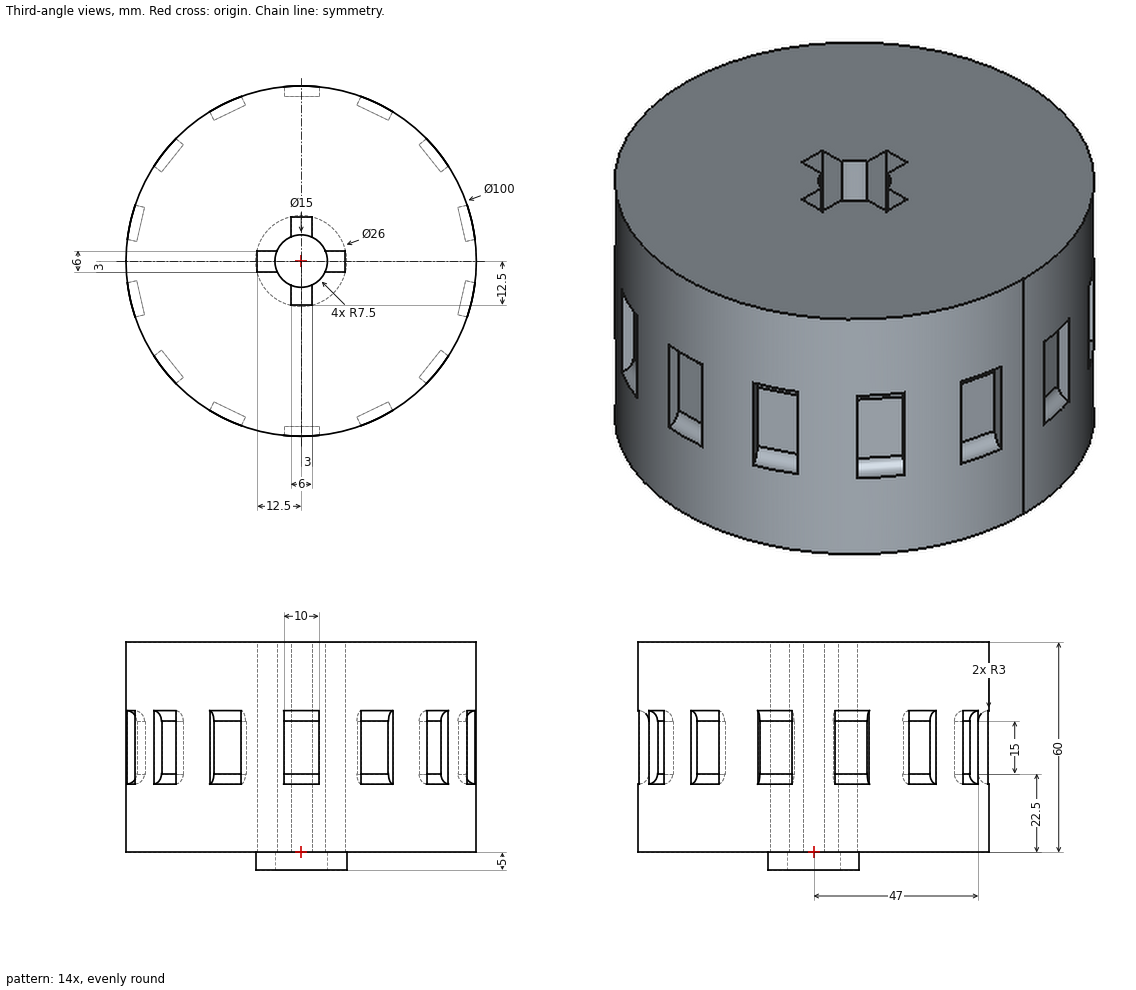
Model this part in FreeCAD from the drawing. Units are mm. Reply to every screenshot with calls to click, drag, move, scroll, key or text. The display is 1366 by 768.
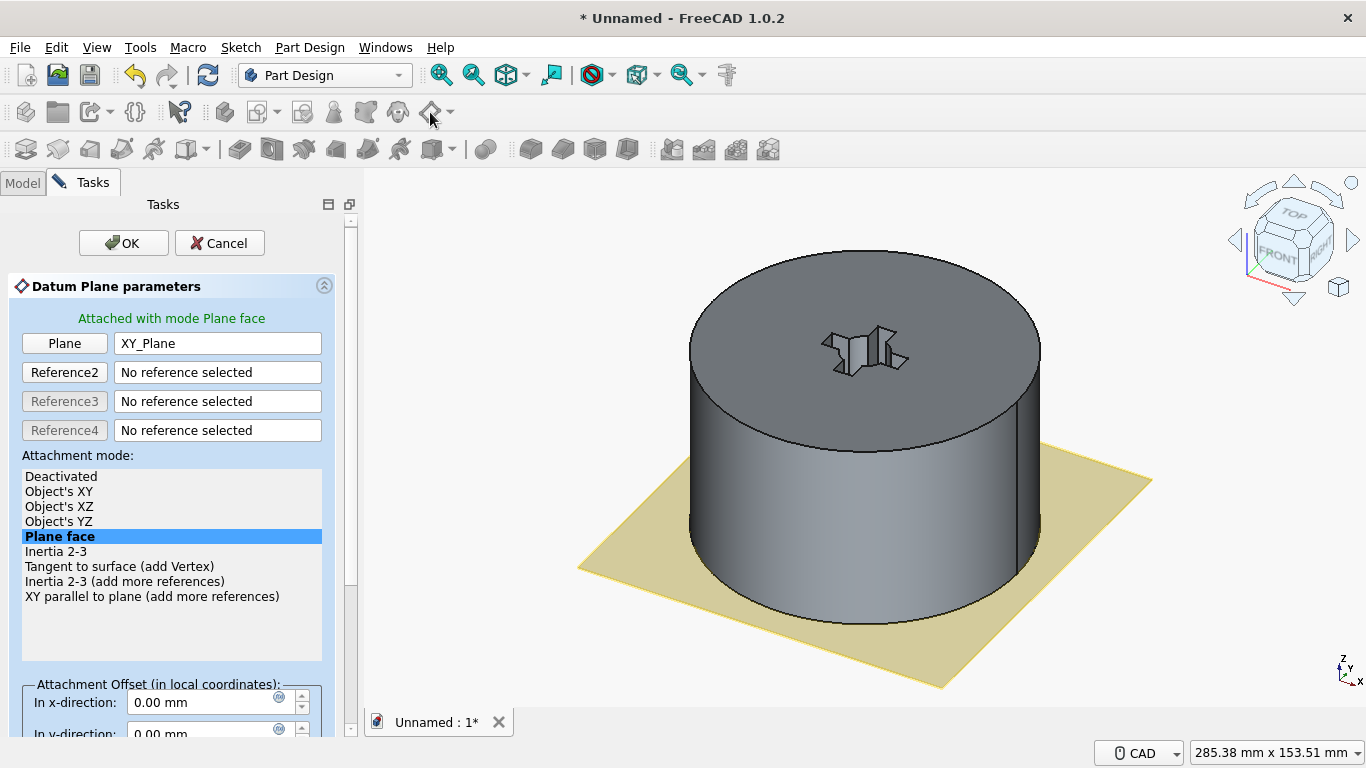
scroll(351, 475, down, 2)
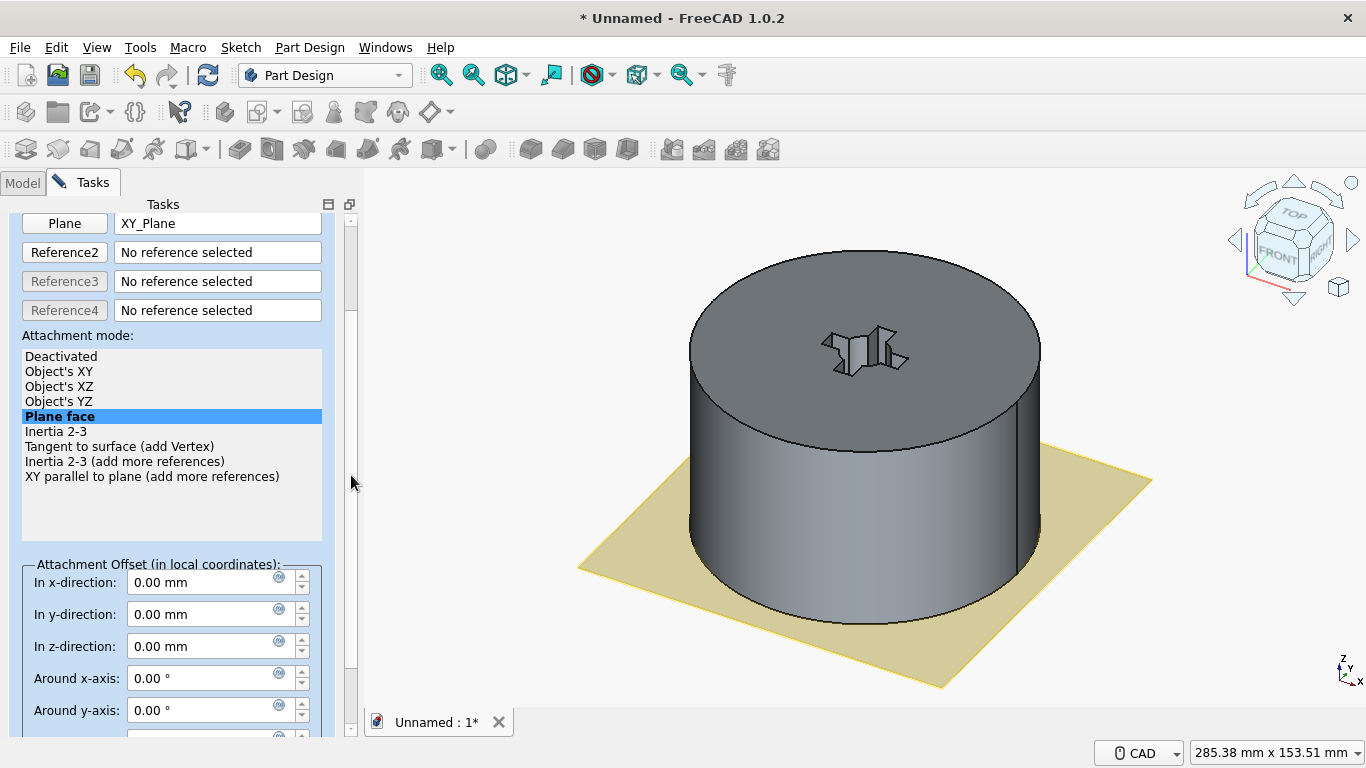
triple_click(210, 646)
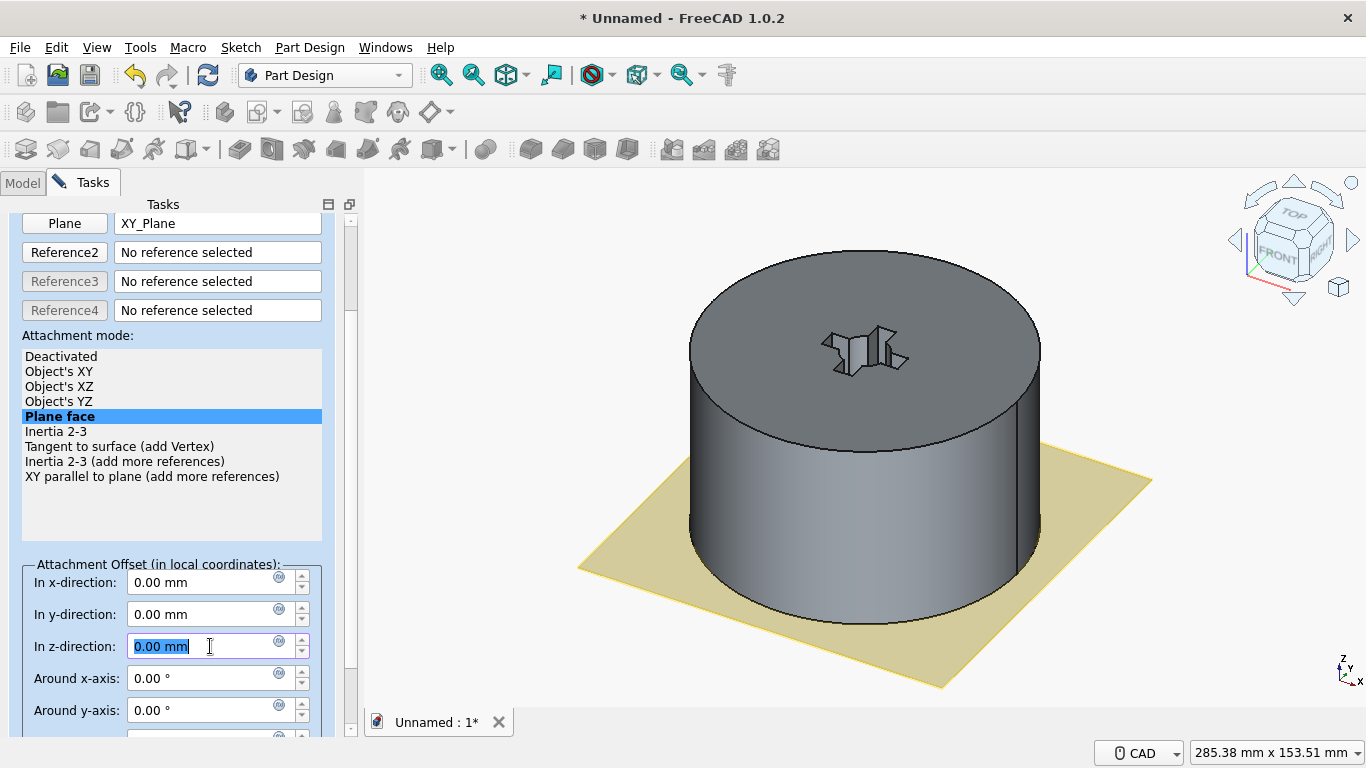
text(-5)
key(Tab)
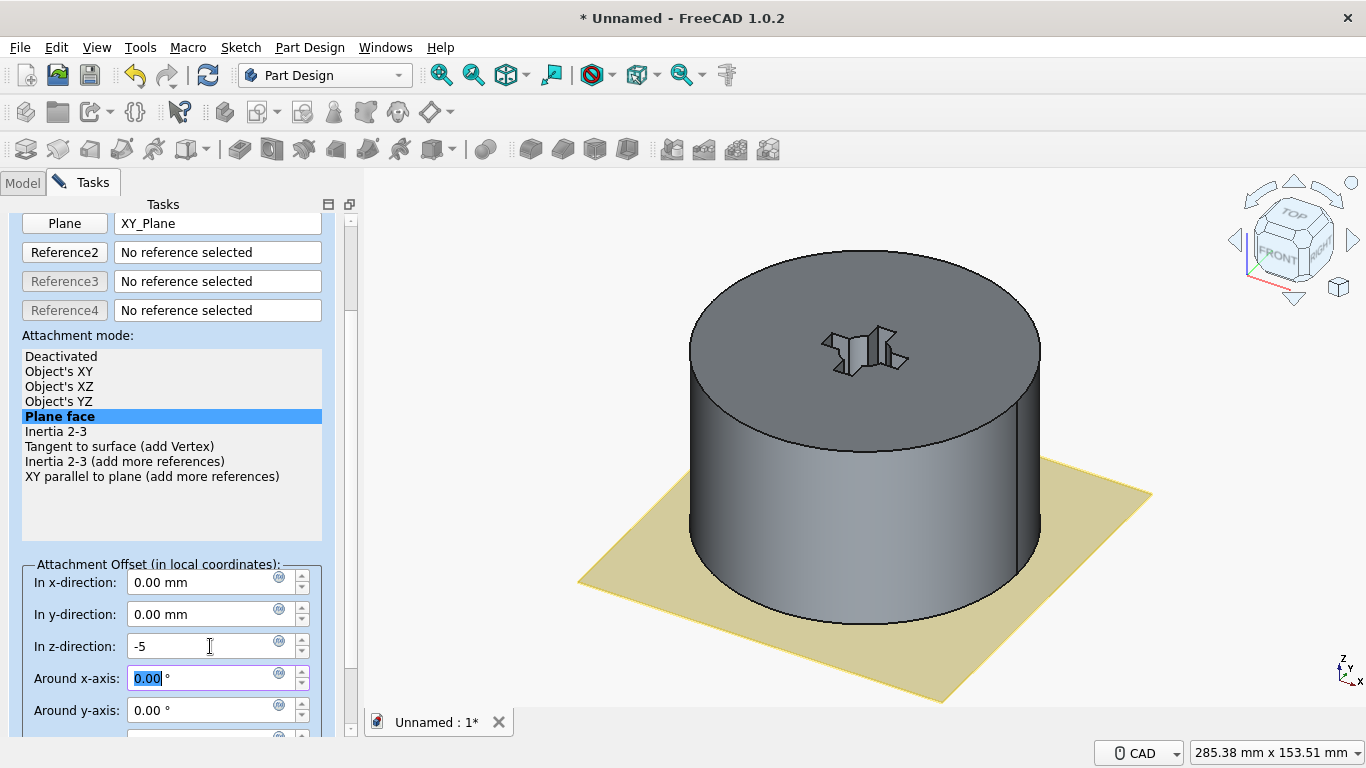
scroll(351, 475, up, 3)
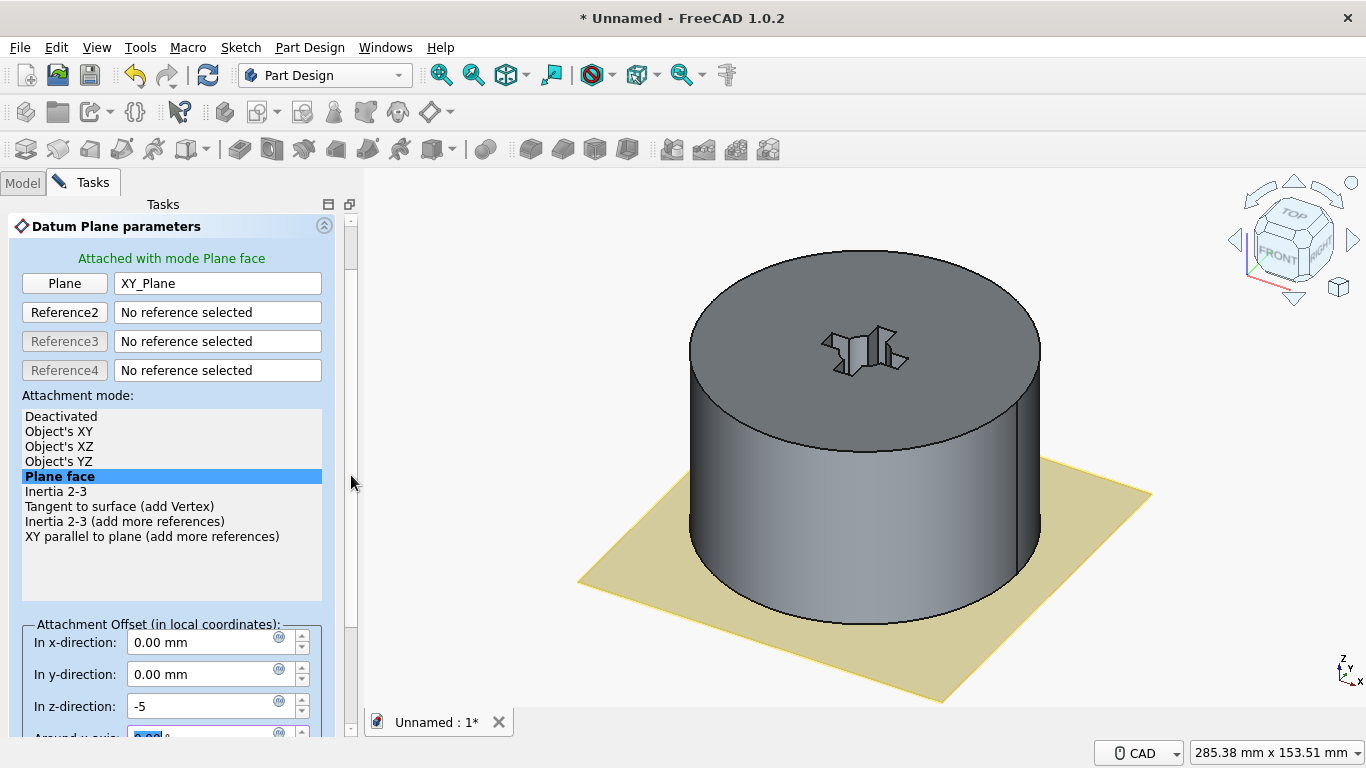
click(124, 243)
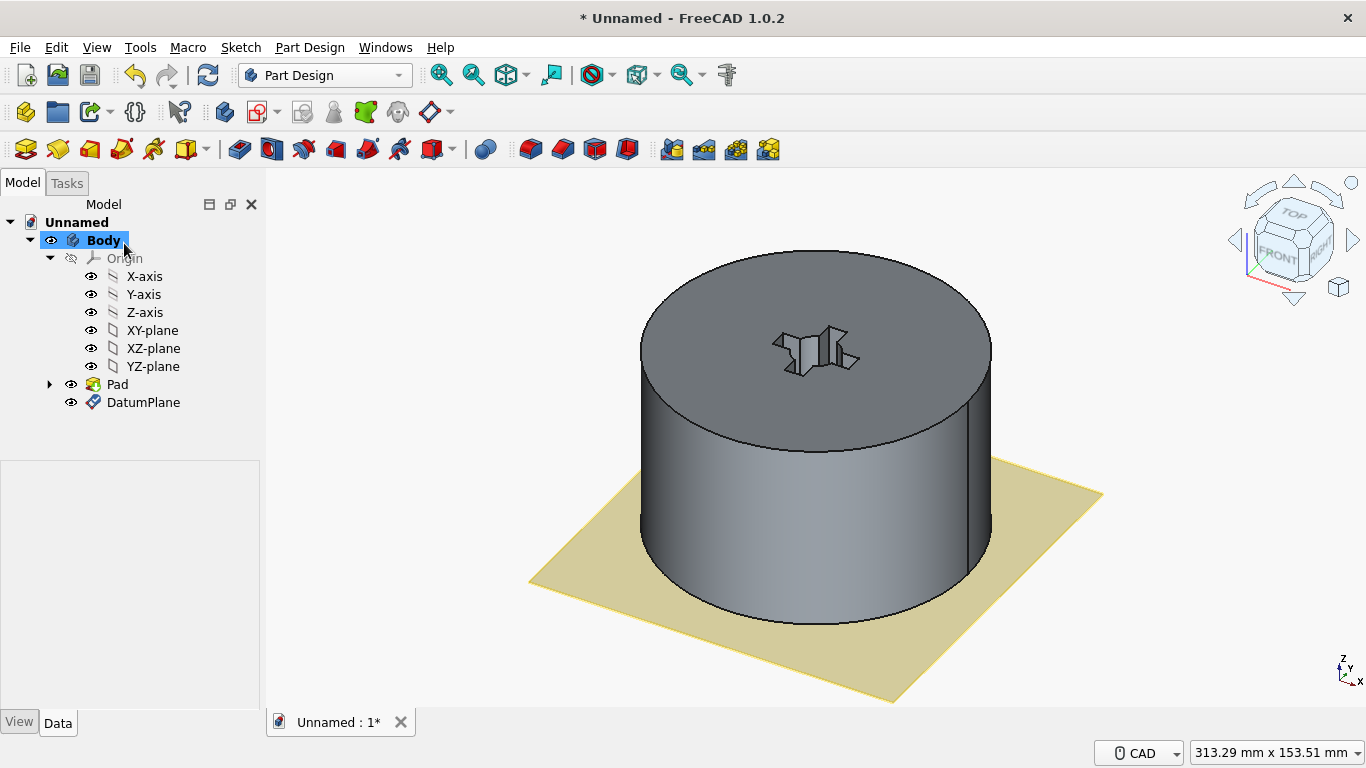
click(116, 402)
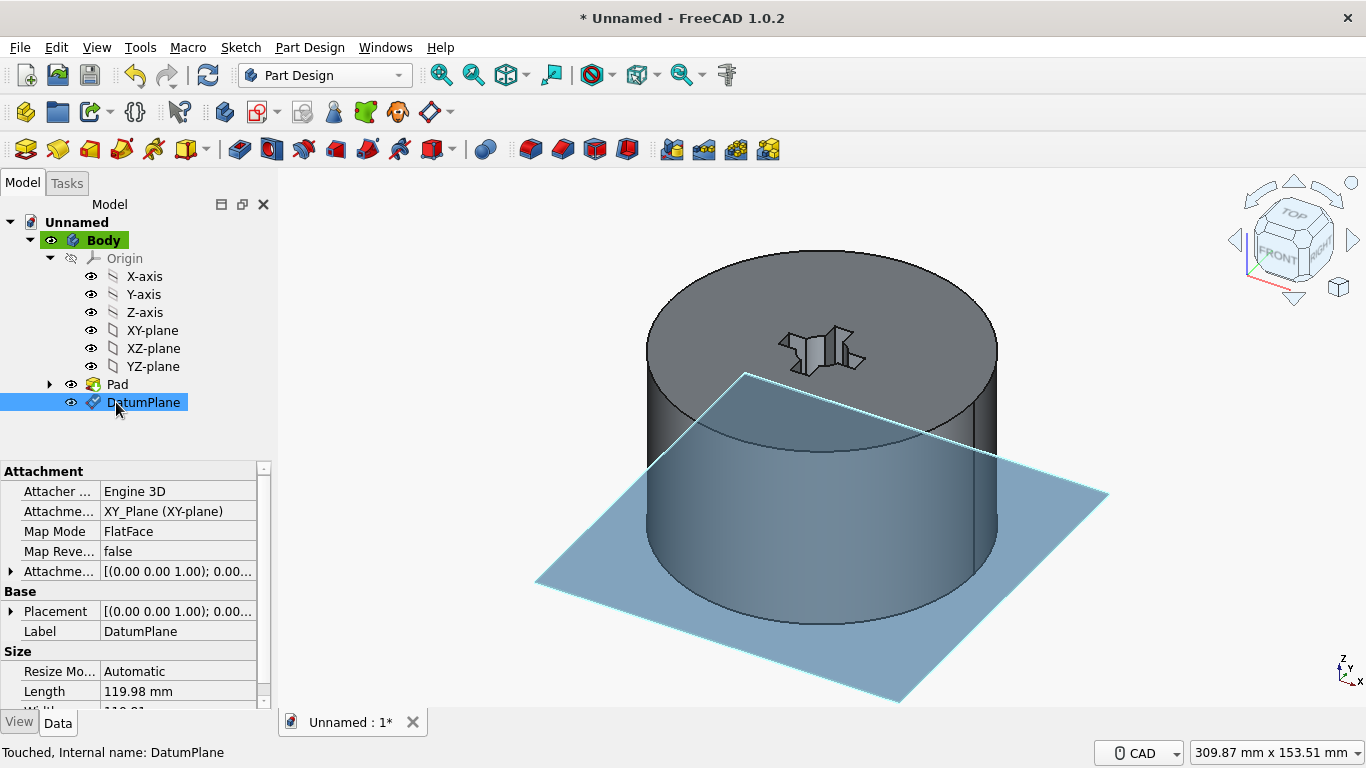
click(258, 112)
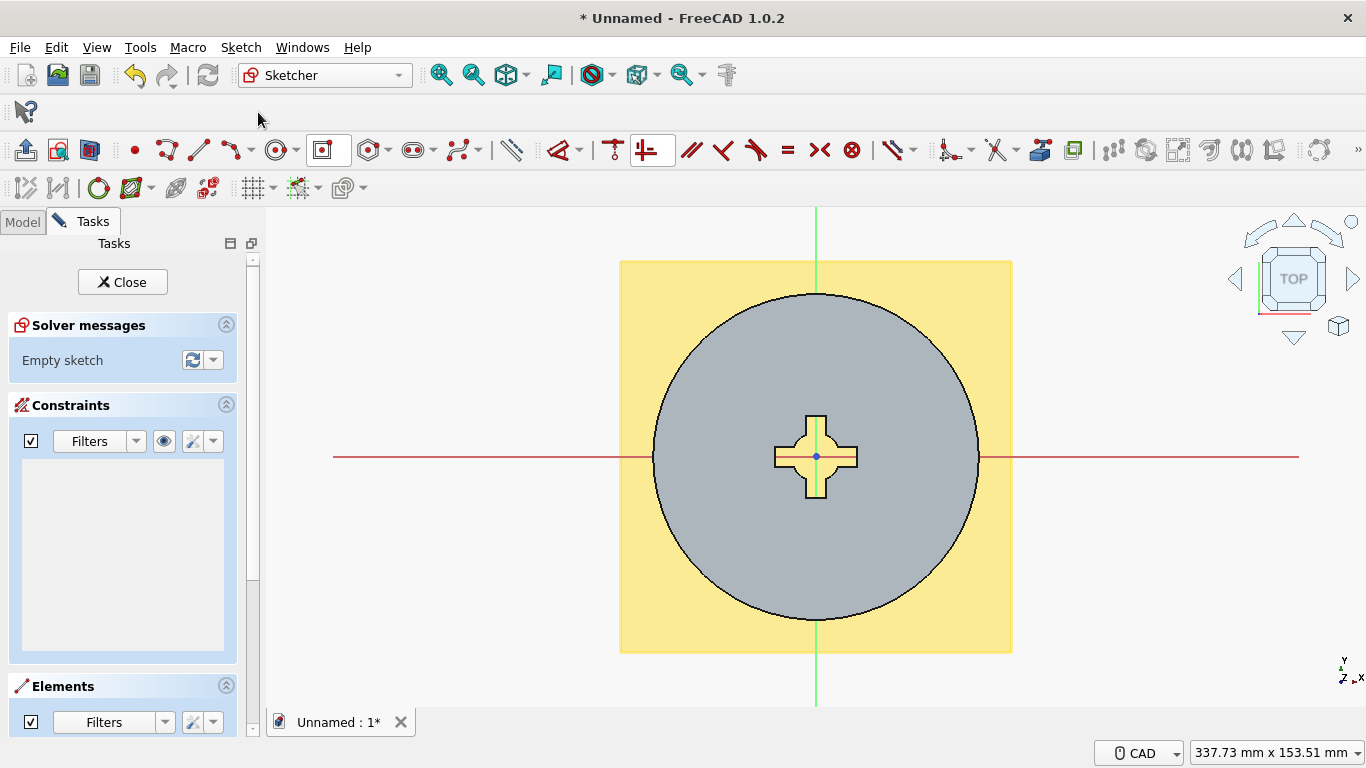
click(90, 150)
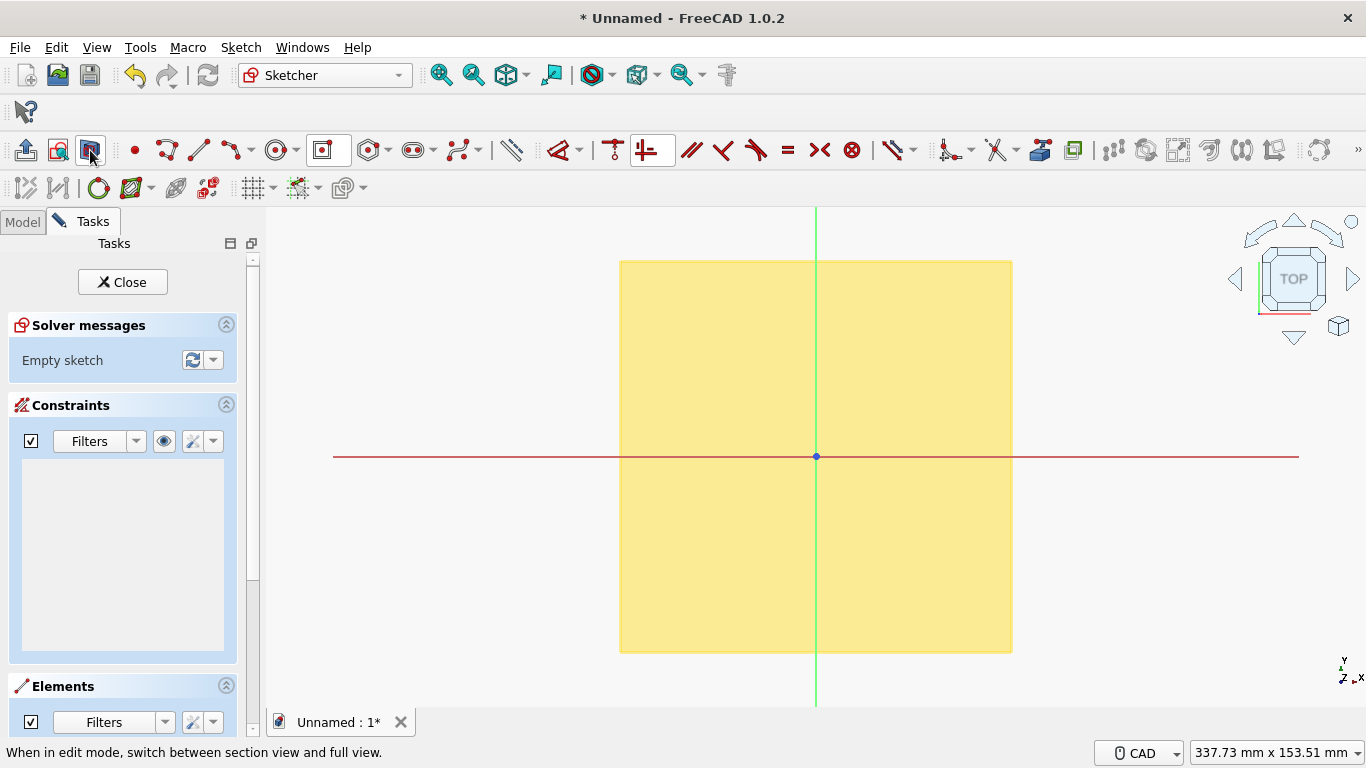
scroll(838, 457, up, 7)